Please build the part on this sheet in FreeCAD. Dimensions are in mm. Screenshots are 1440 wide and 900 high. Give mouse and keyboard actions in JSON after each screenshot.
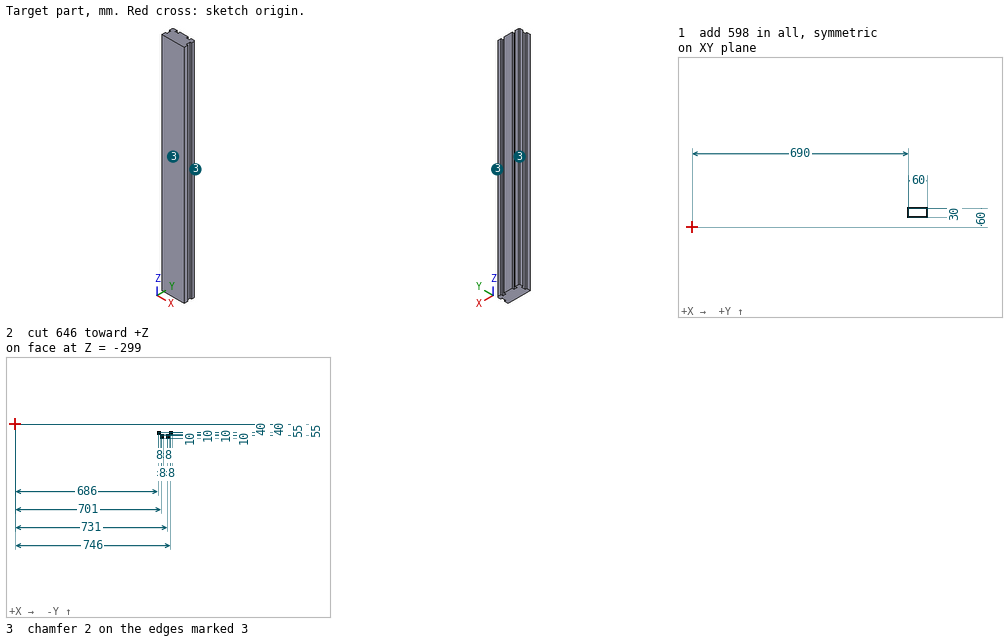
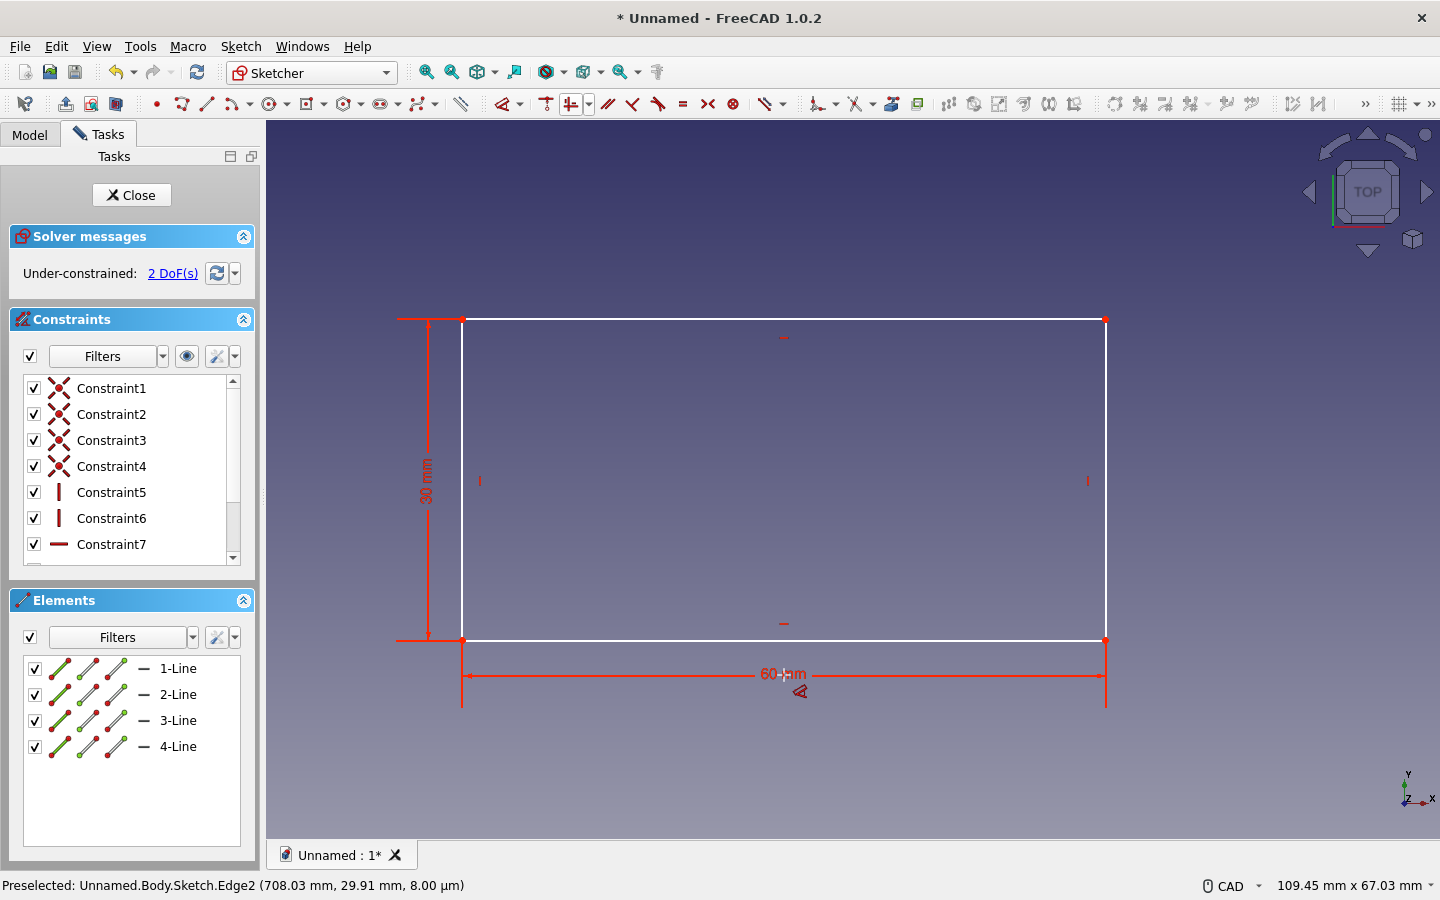
{"action": "left_click", "coordinate": [462, 319]}
{"action": "left_click", "coordinate": [496, 565]}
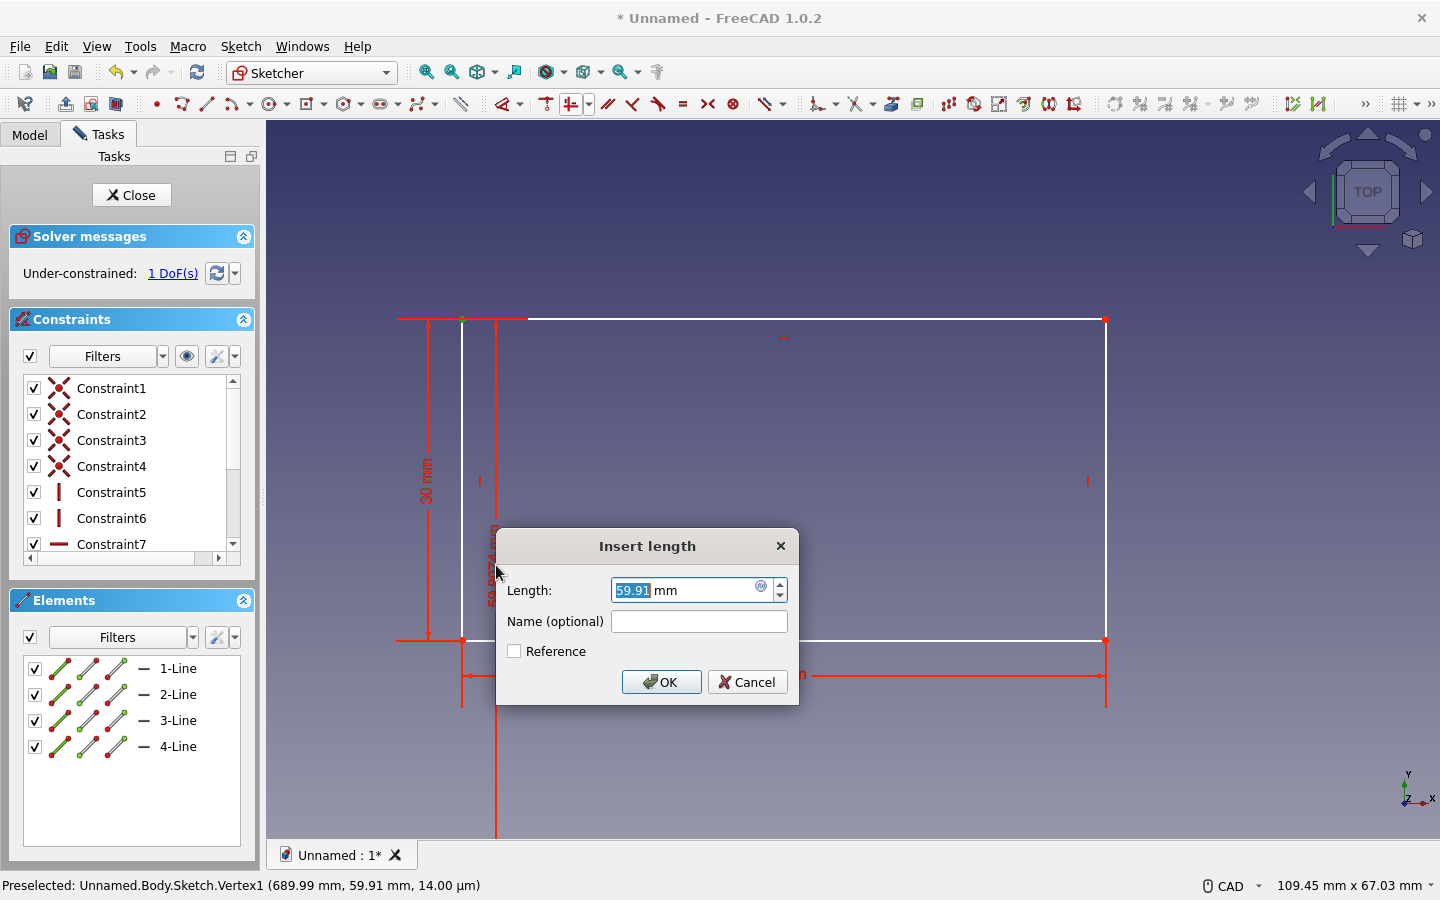
{"action": "type", "text": "60"}
{"action": "key", "text": "Return"}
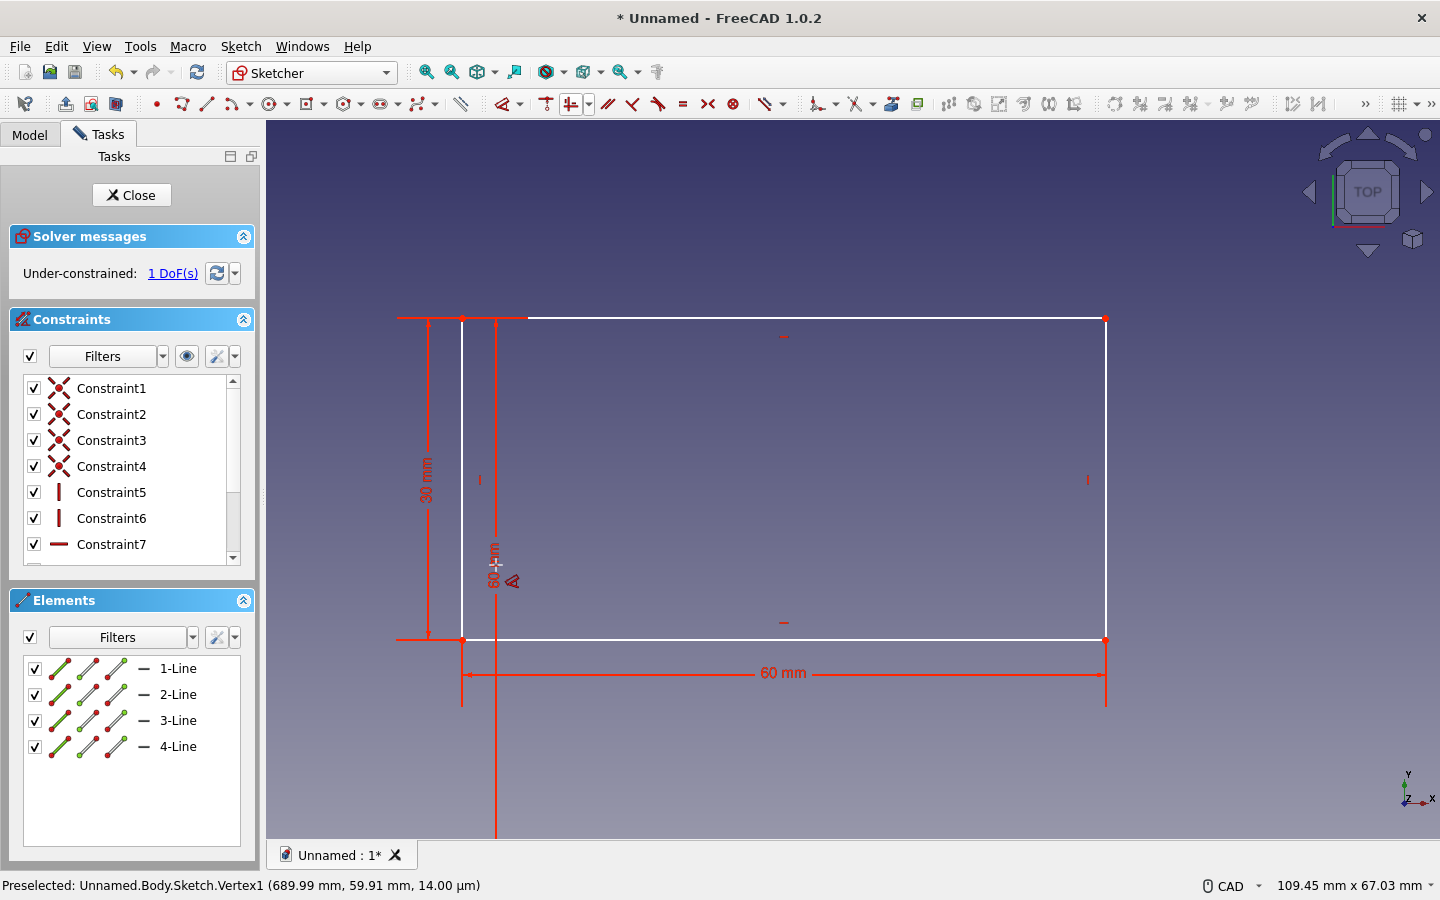
{"action": "left_click", "coordinate": [462, 318]}
{"action": "left_click", "coordinate": [378, 284]}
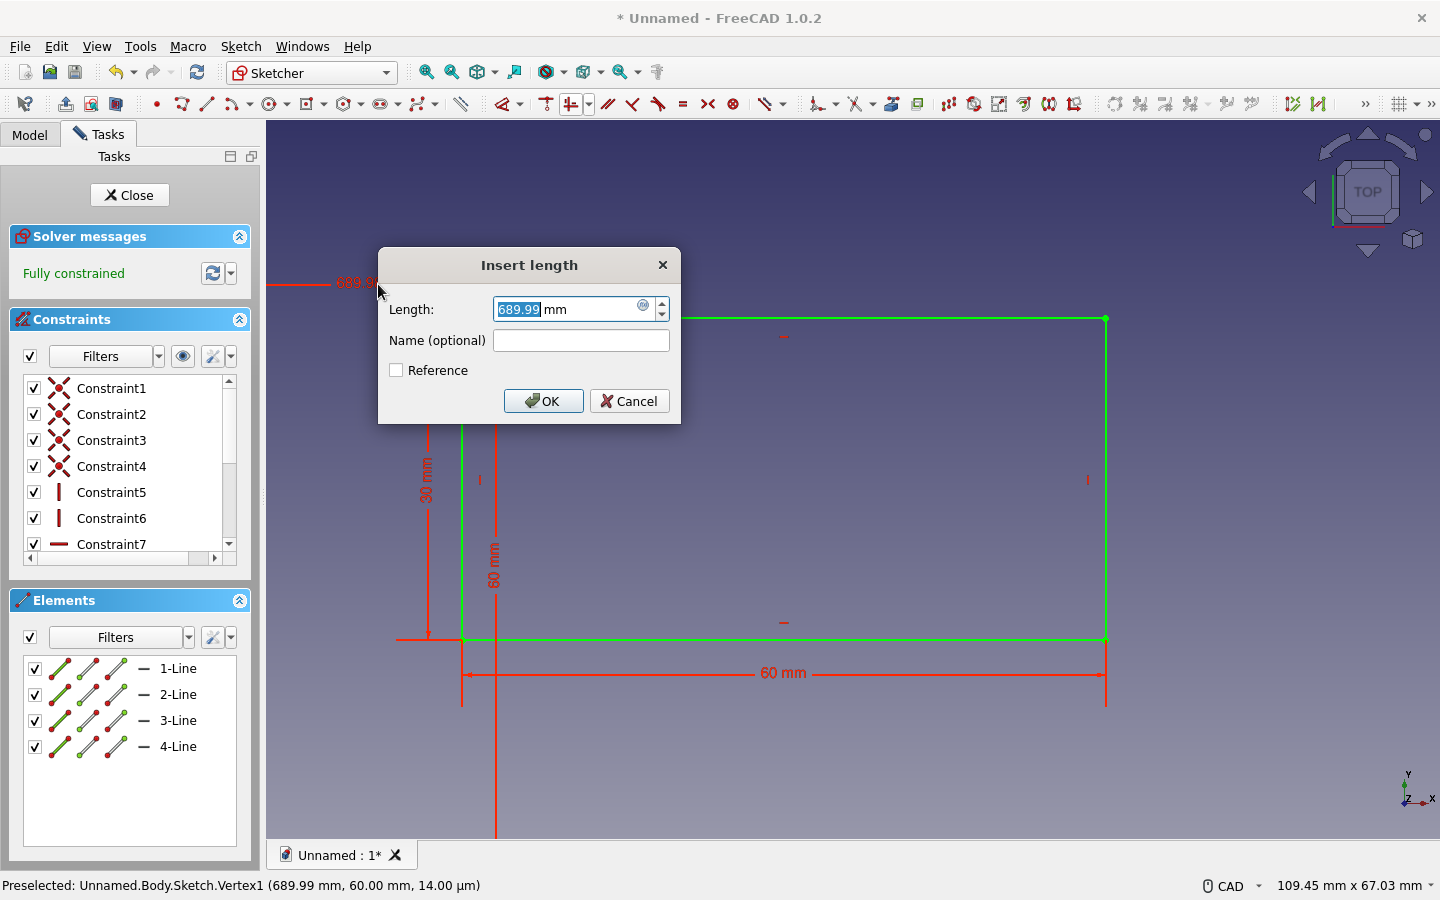
{"action": "type", "text": "690"}
{"action": "key", "text": "Return"}
{"action": "key", "text": "Escape"}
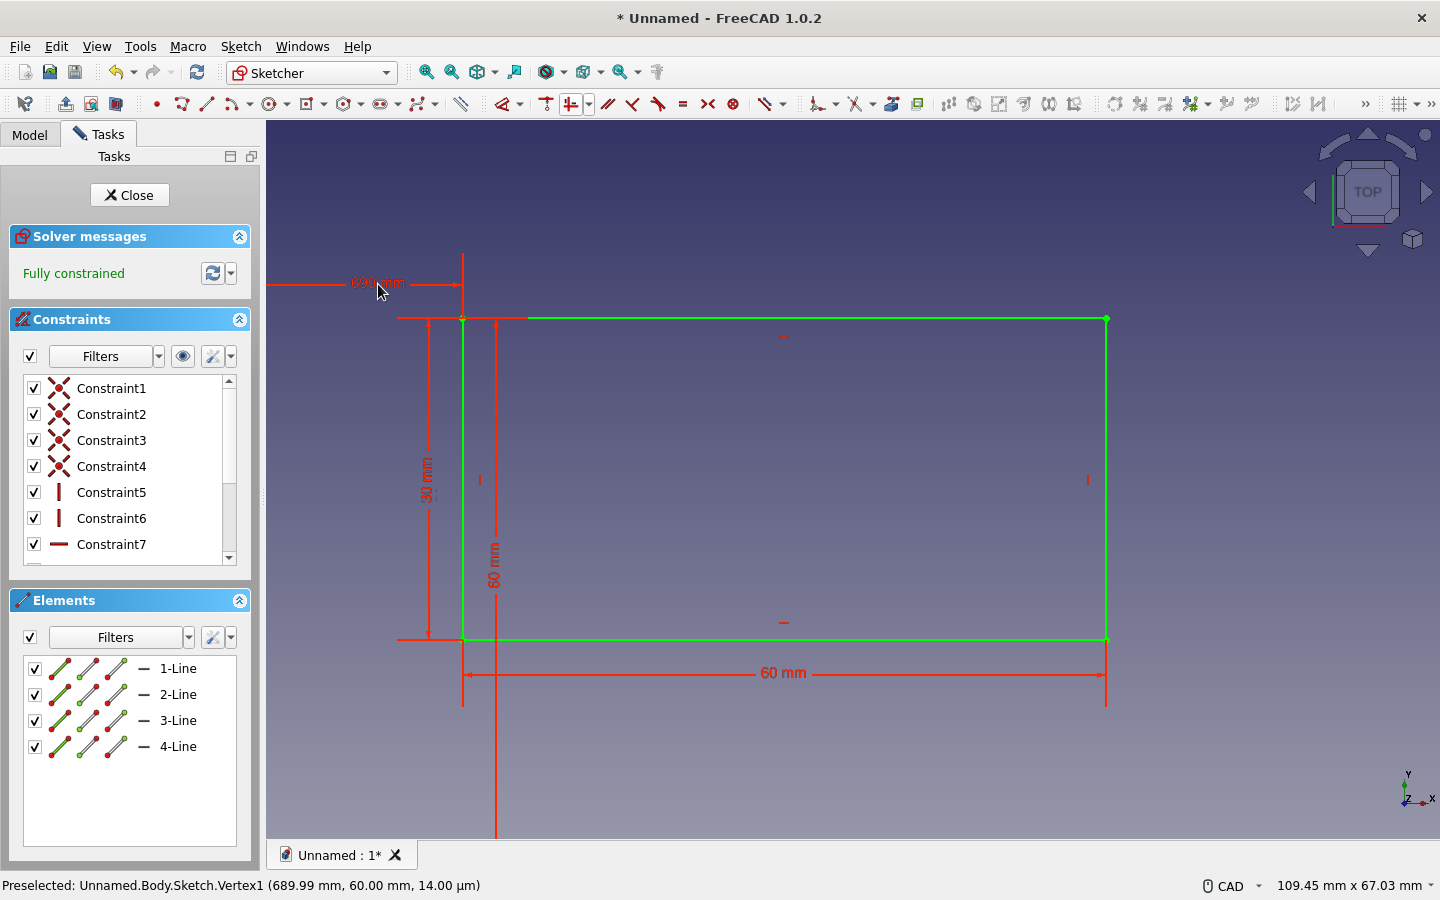
{"action": "left_click", "coordinate": [130, 195]}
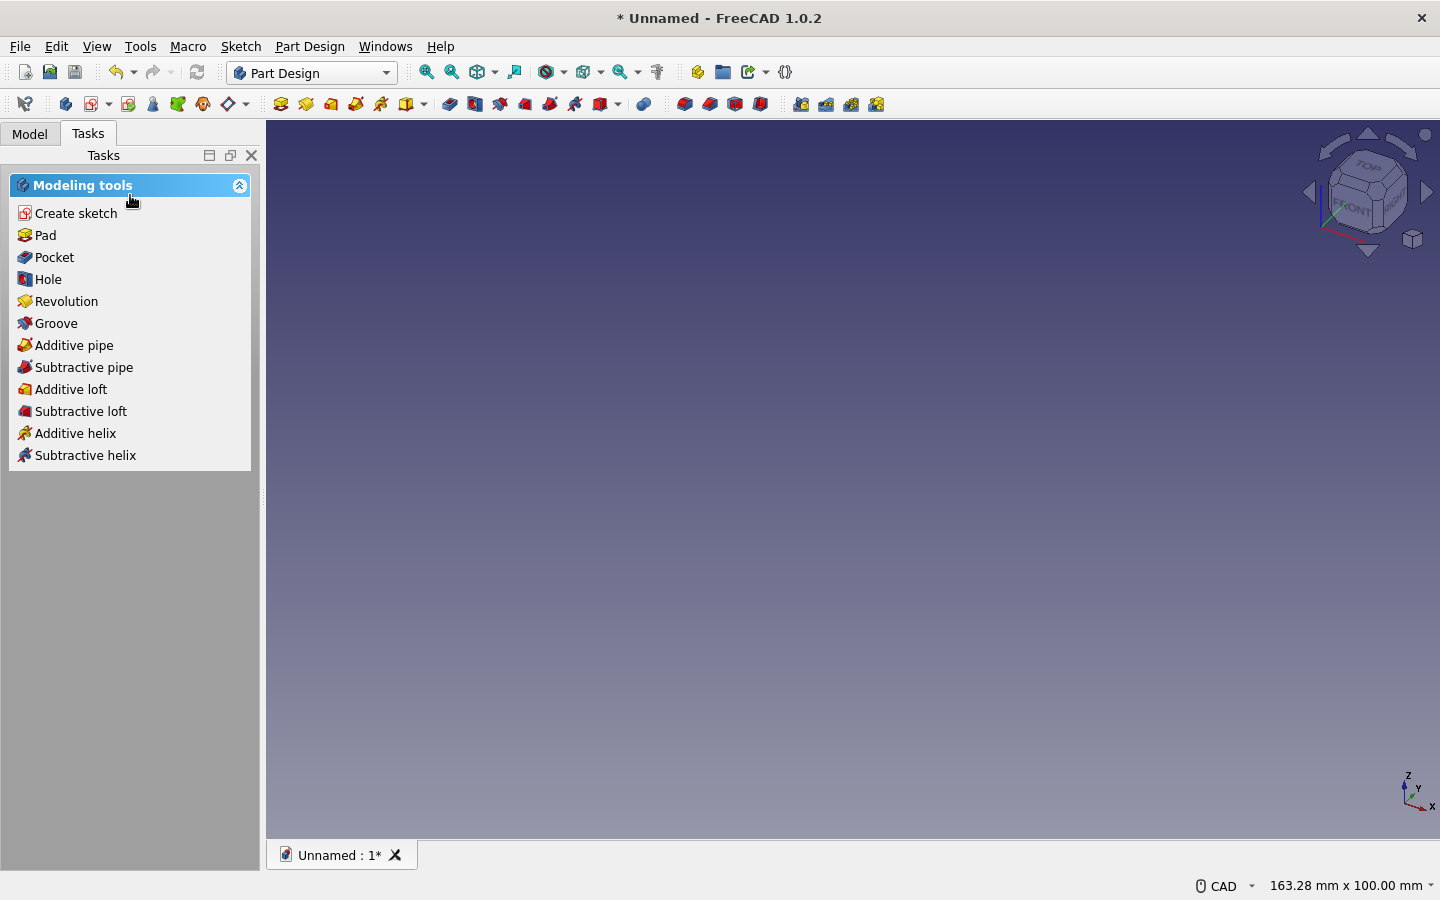
{"action": "left_click", "coordinate": [281, 104]}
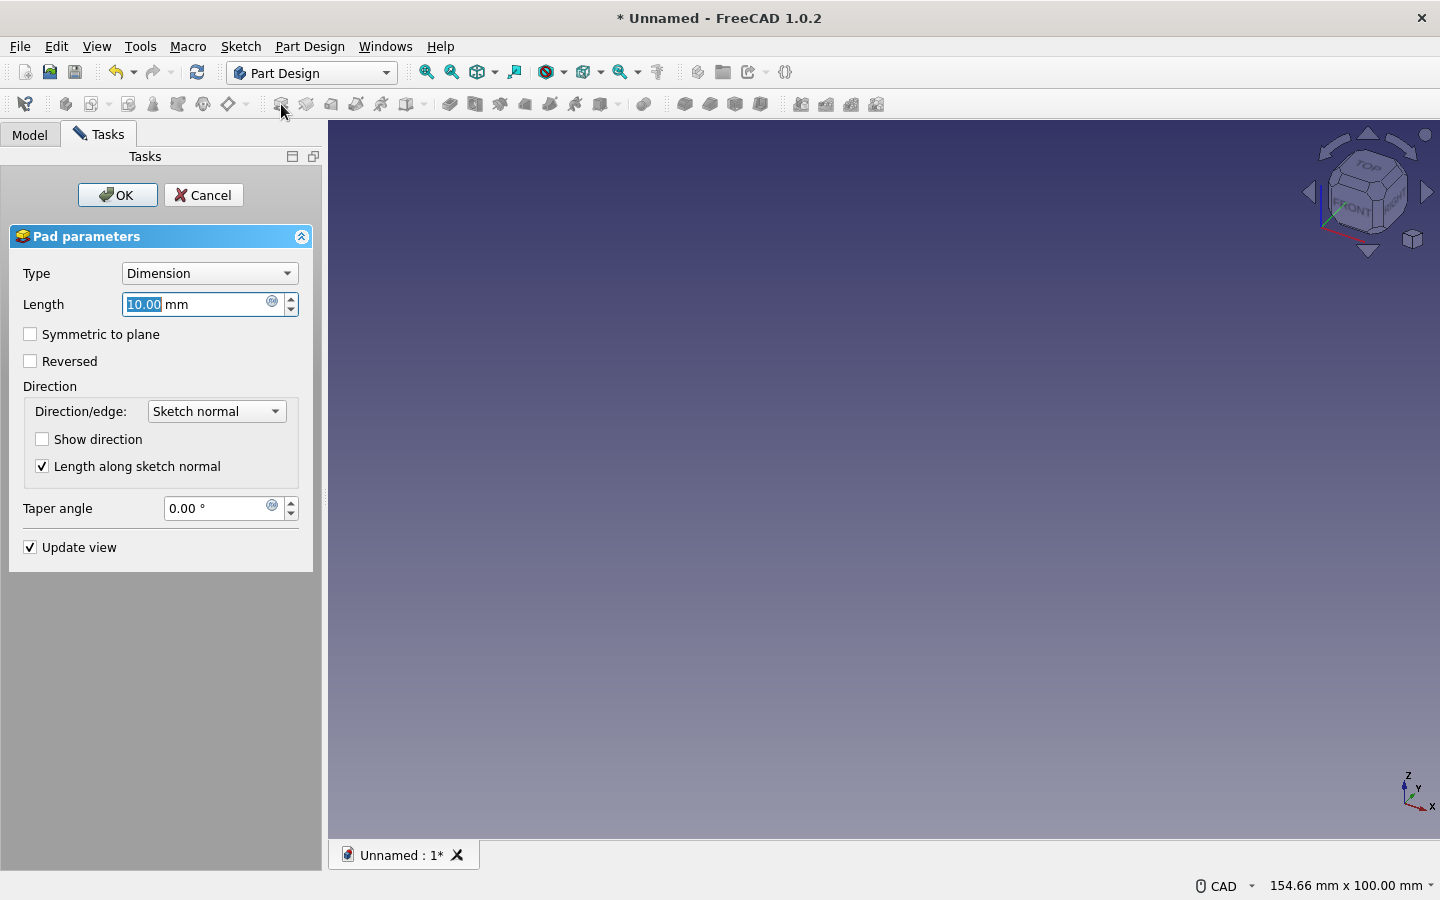
{"action": "type", "text": "598"}
{"action": "key", "text": "Tab"}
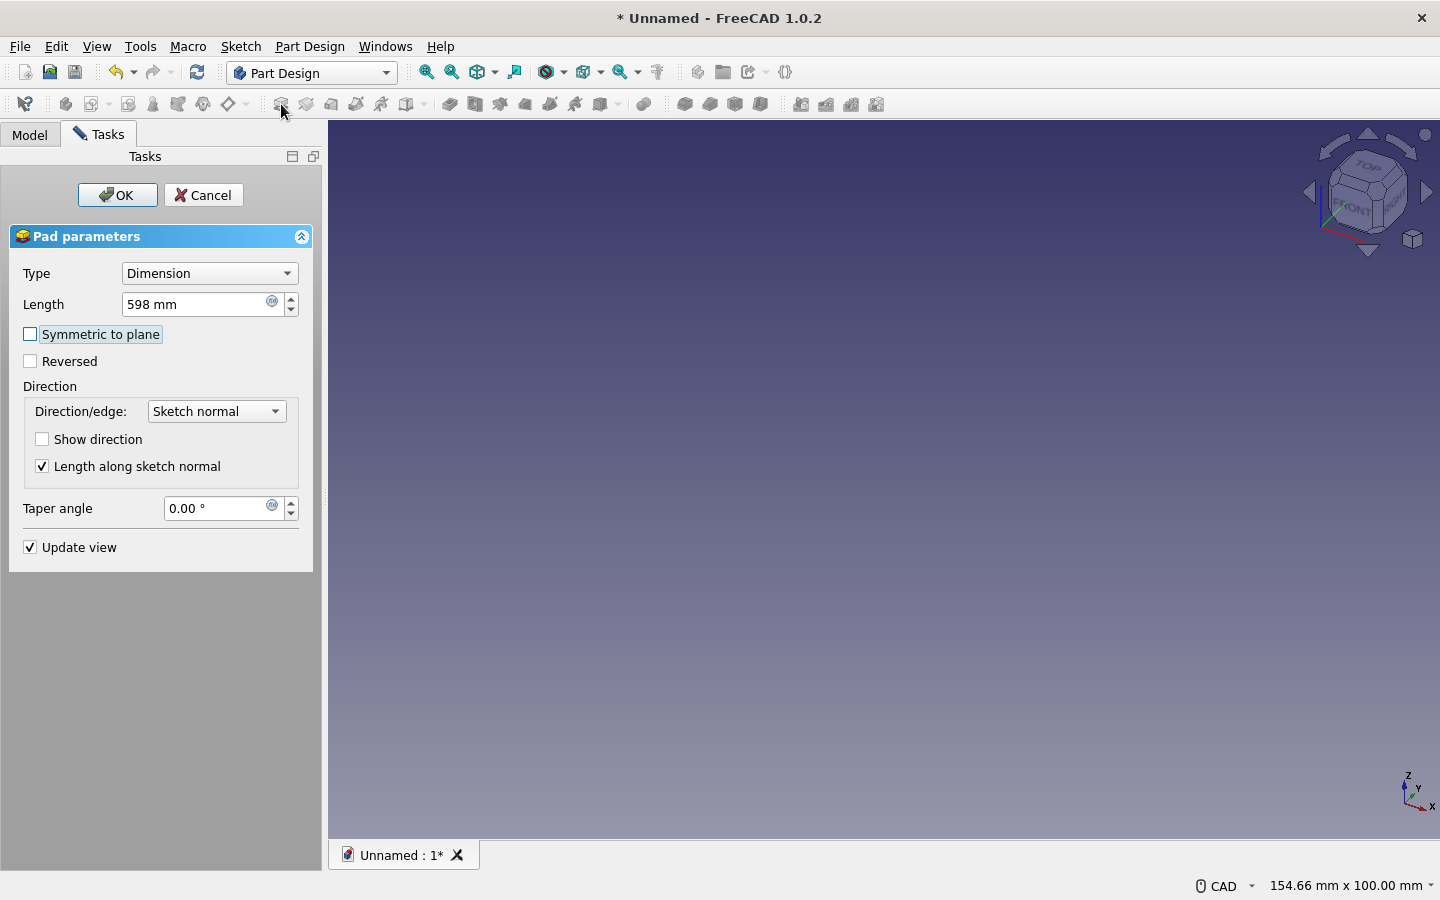
{"action": "left_click", "coordinate": [31, 334]}